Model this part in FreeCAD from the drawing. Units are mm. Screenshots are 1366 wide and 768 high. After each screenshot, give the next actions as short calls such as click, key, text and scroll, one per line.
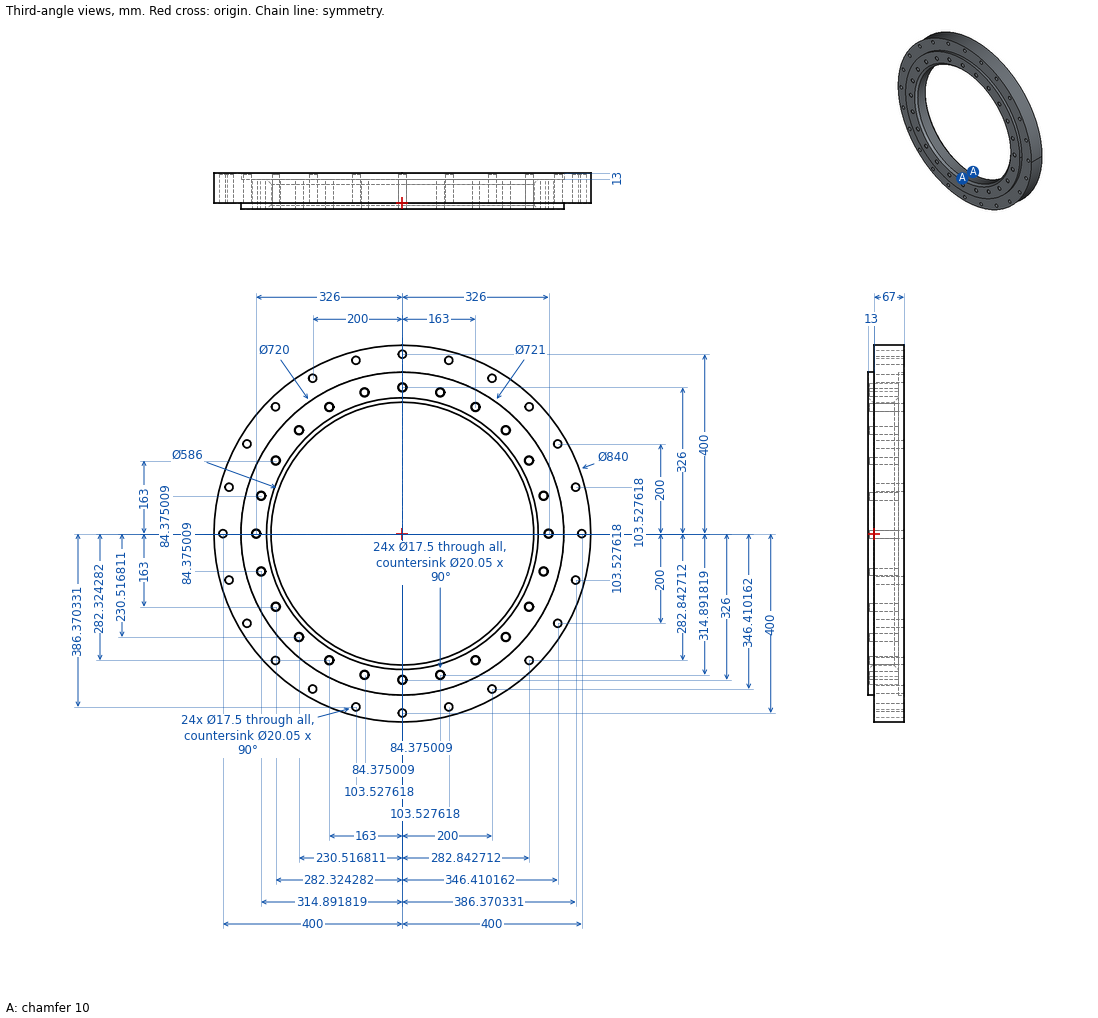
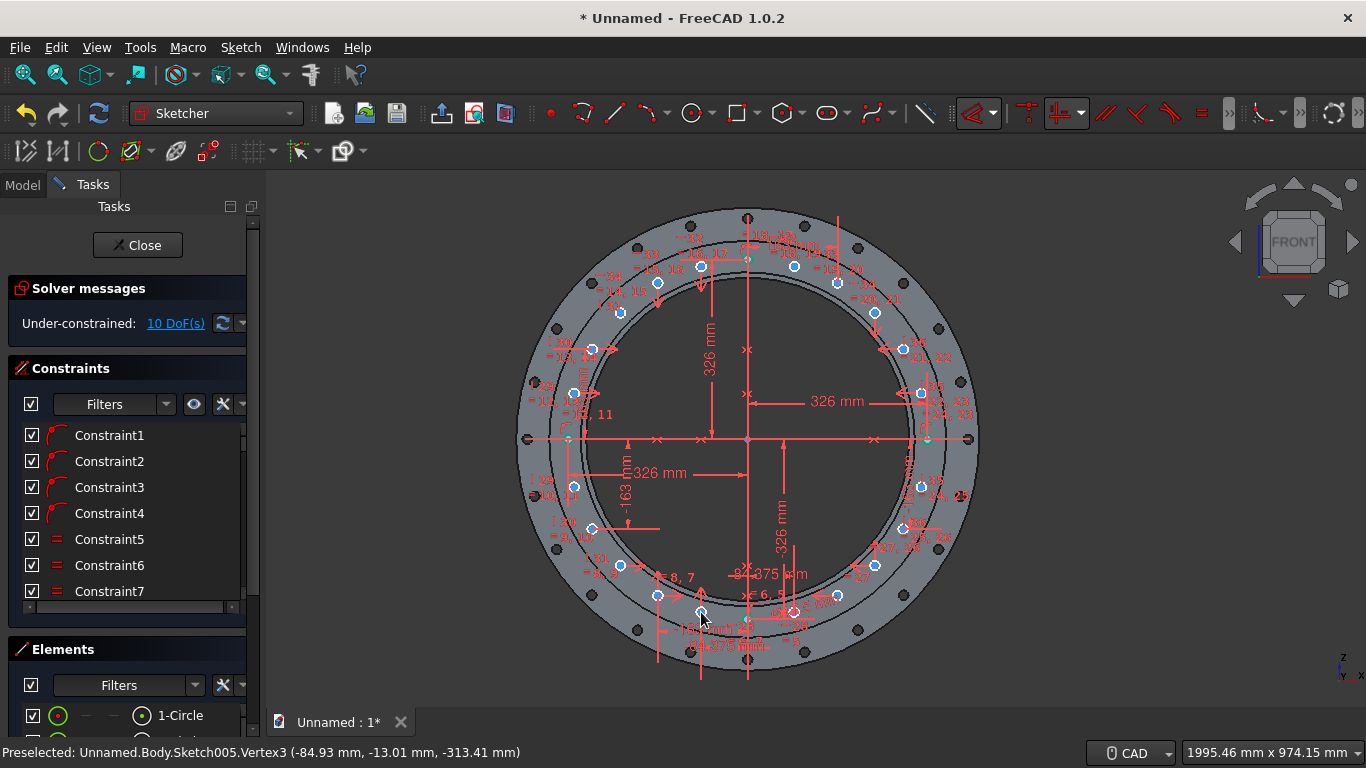
click(574, 487)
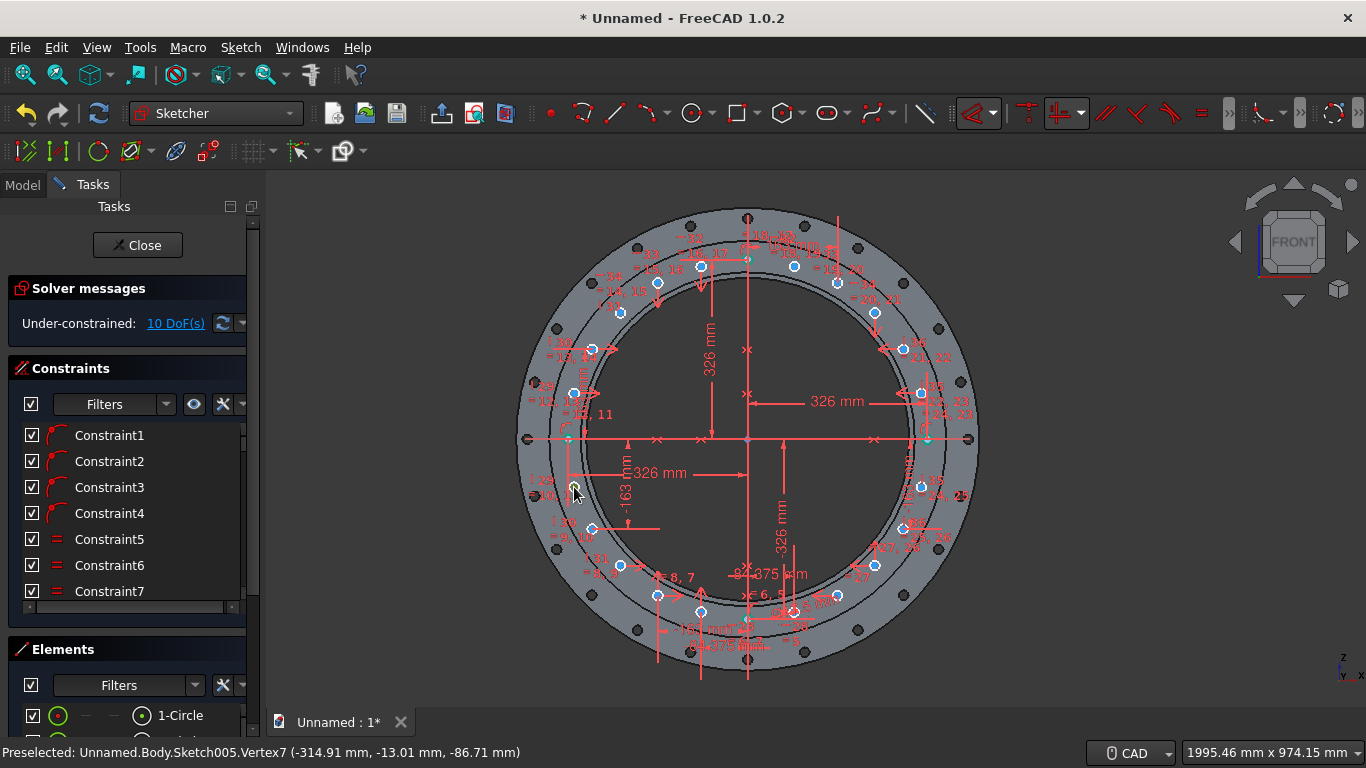
key(i)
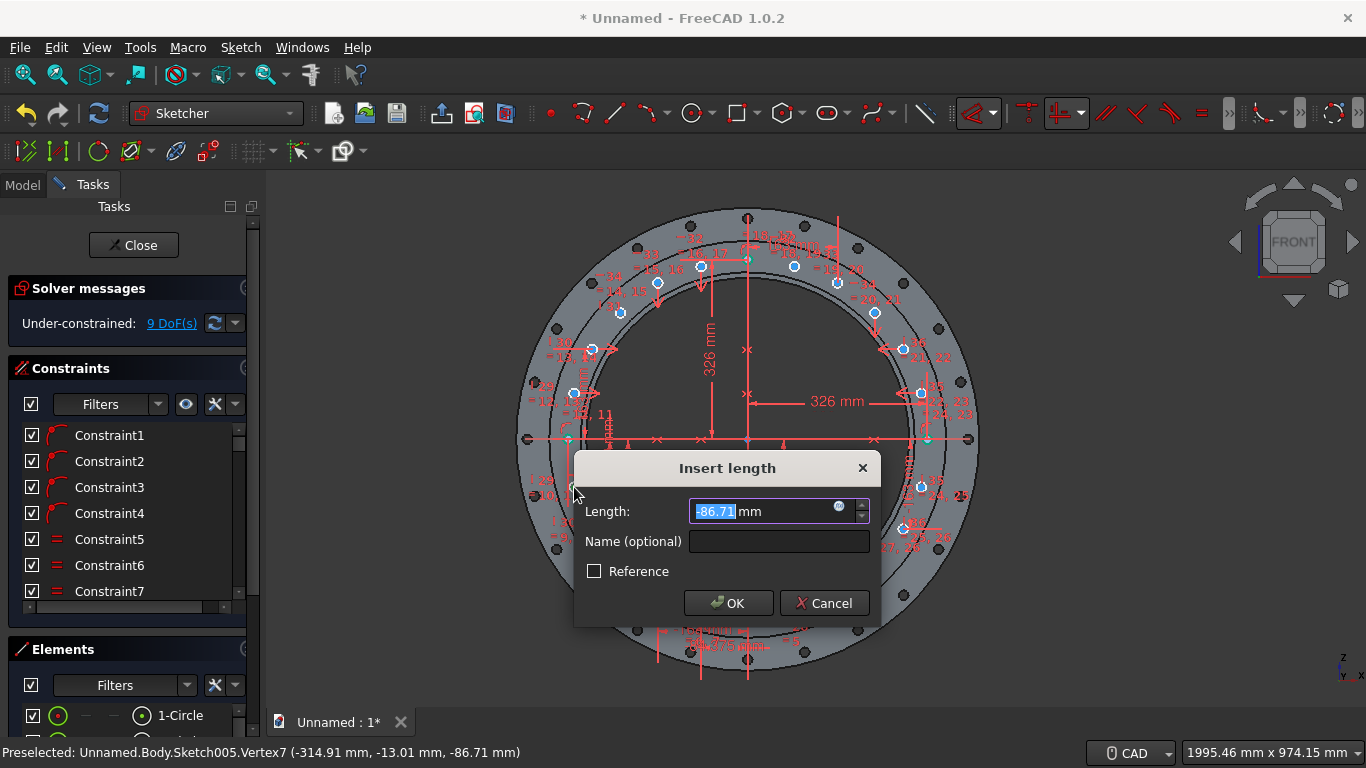
text(-84.375009)
key(Return)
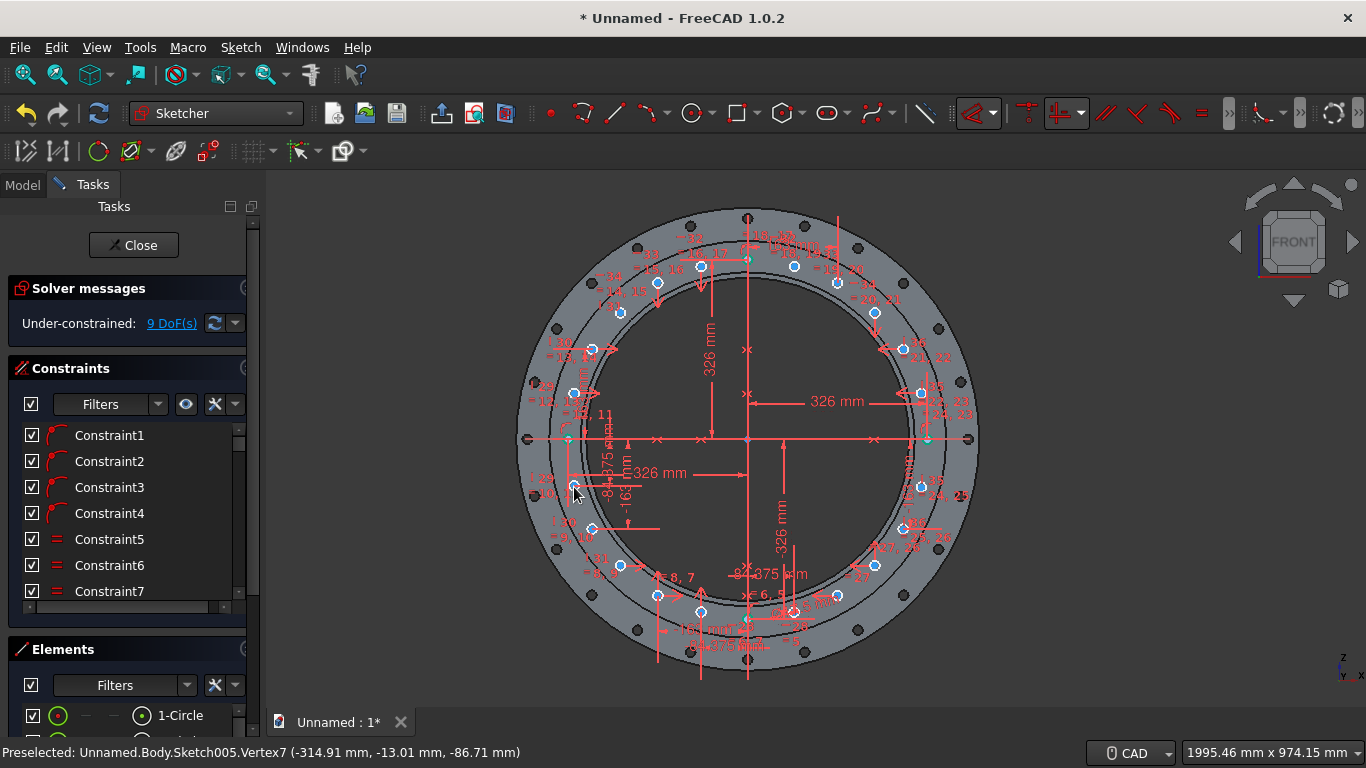
scroll(574, 393, up, 4)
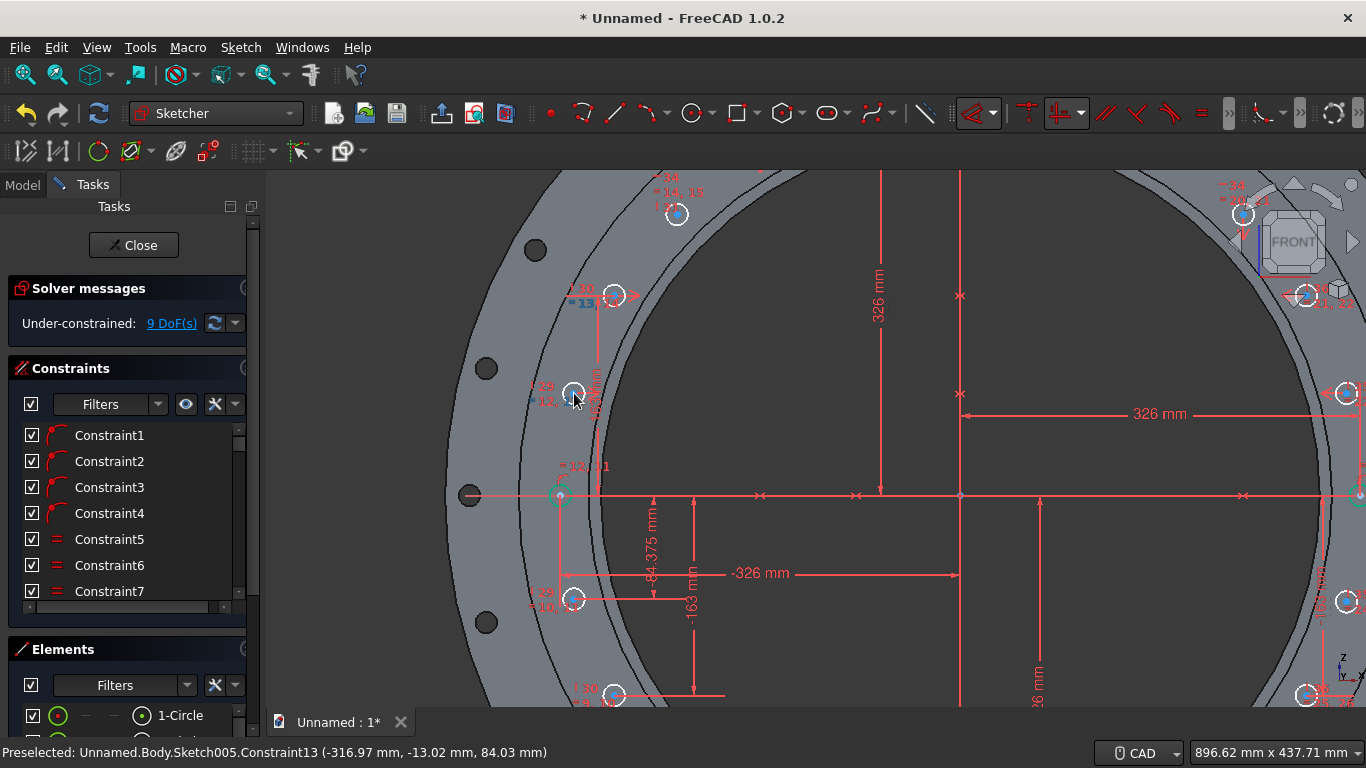
scroll(574, 393, up, 4)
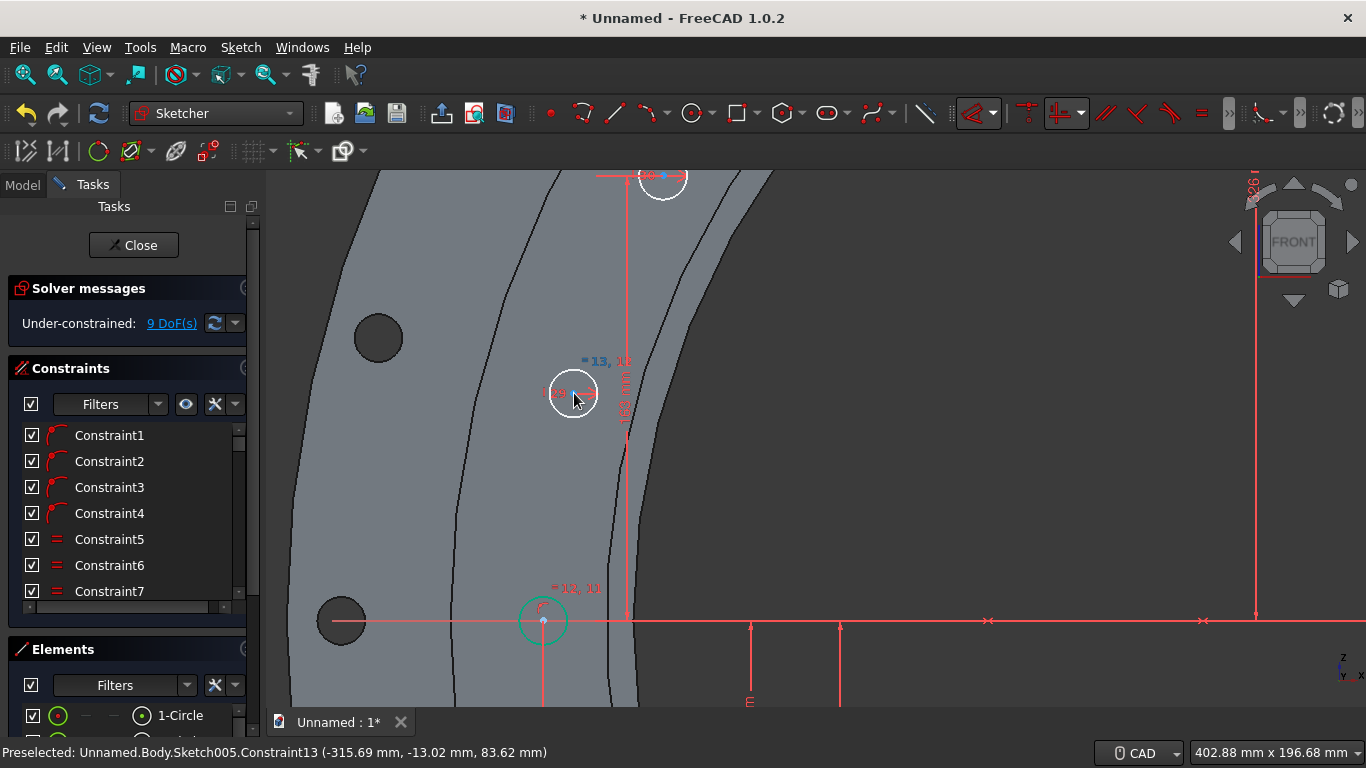
click(574, 394)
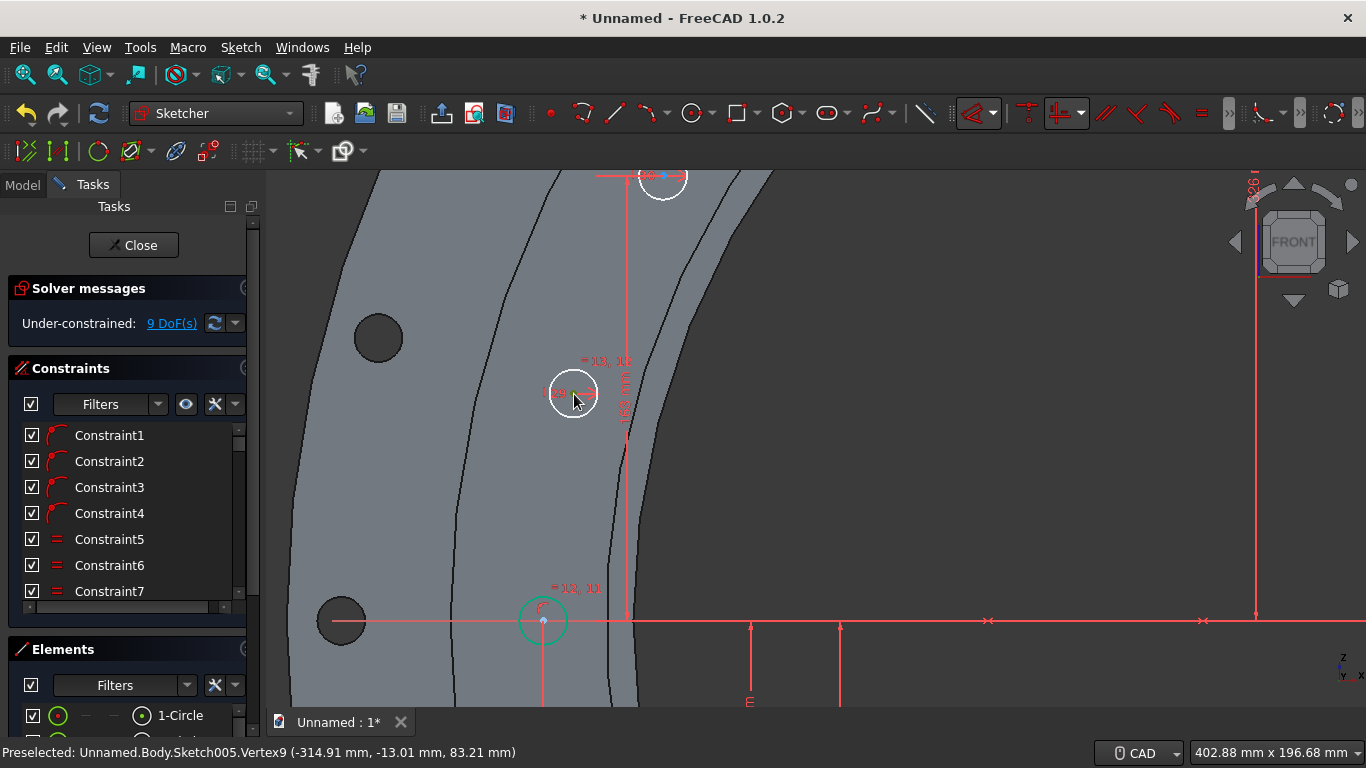
key(i)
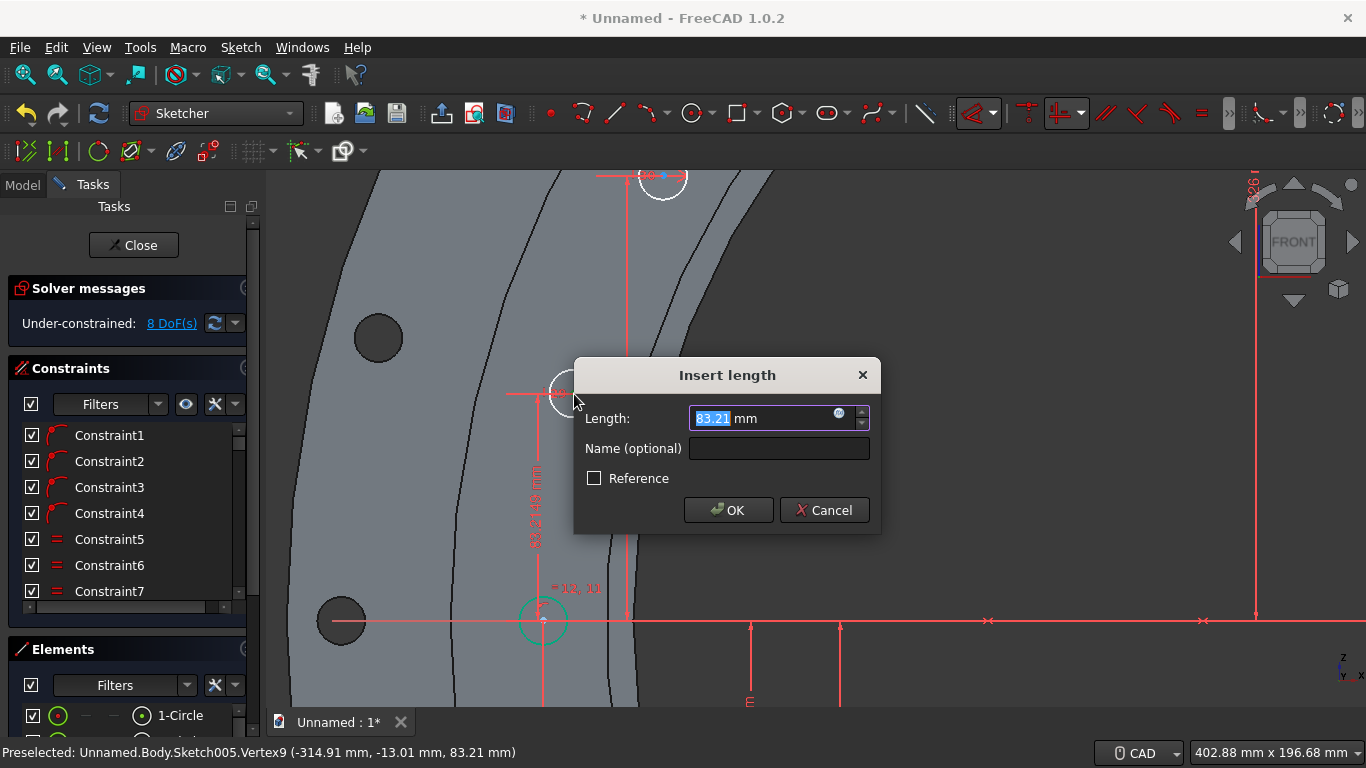
text(84.375009)
key(Return)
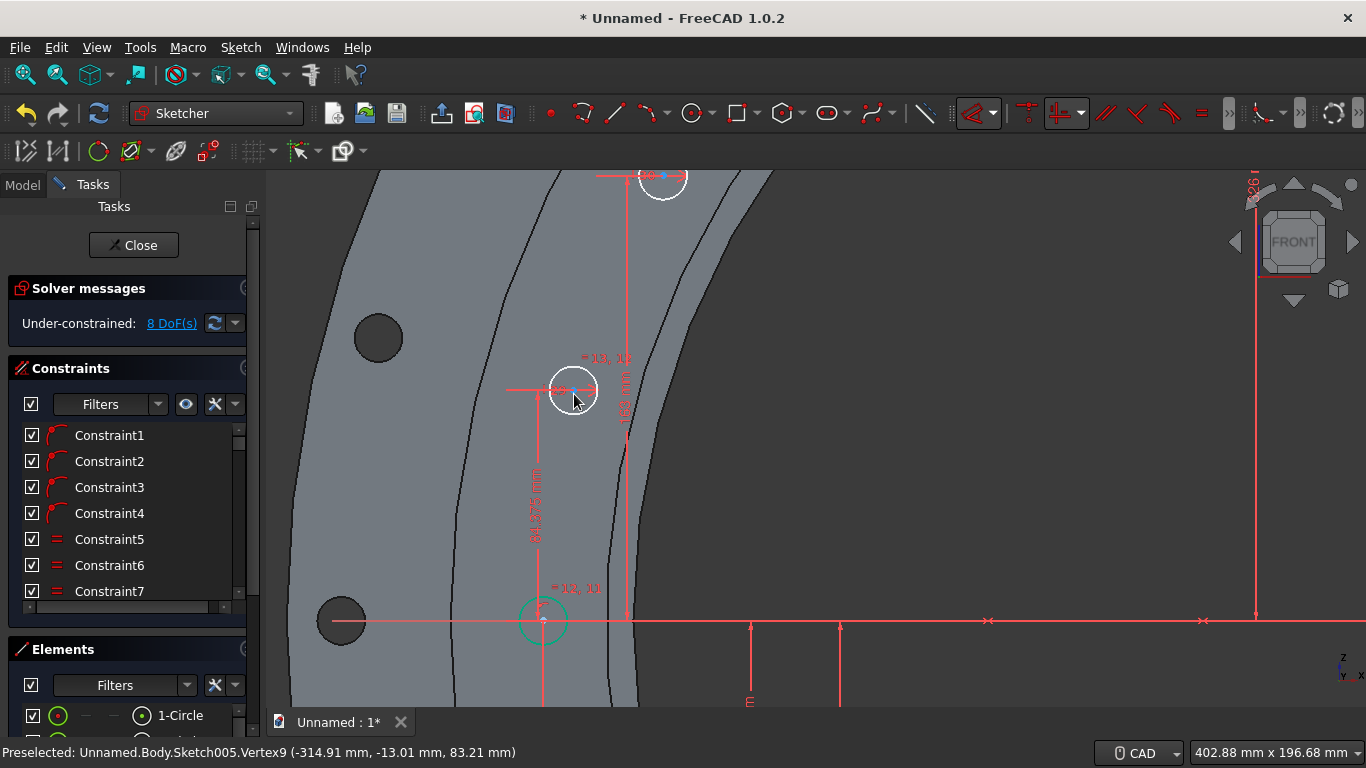
scroll(574, 392, down, 8)